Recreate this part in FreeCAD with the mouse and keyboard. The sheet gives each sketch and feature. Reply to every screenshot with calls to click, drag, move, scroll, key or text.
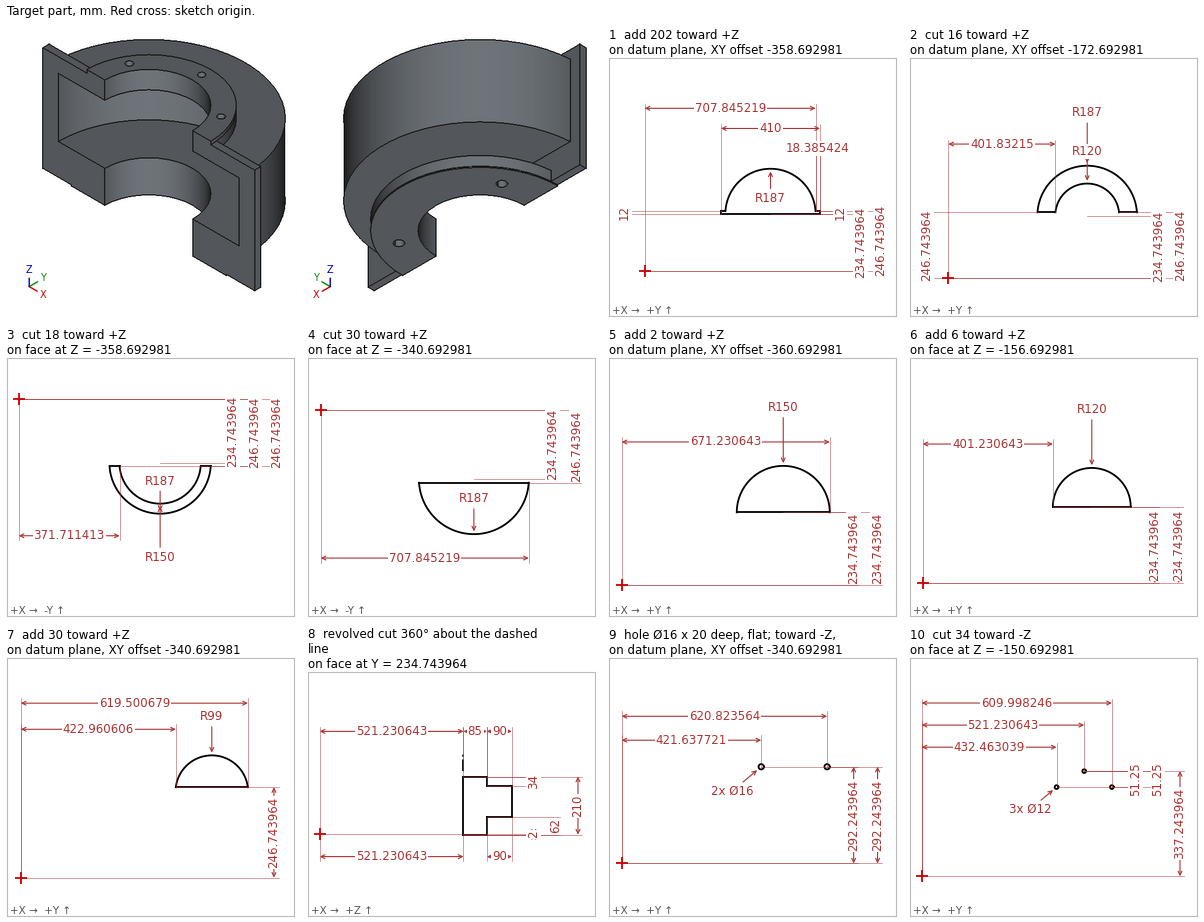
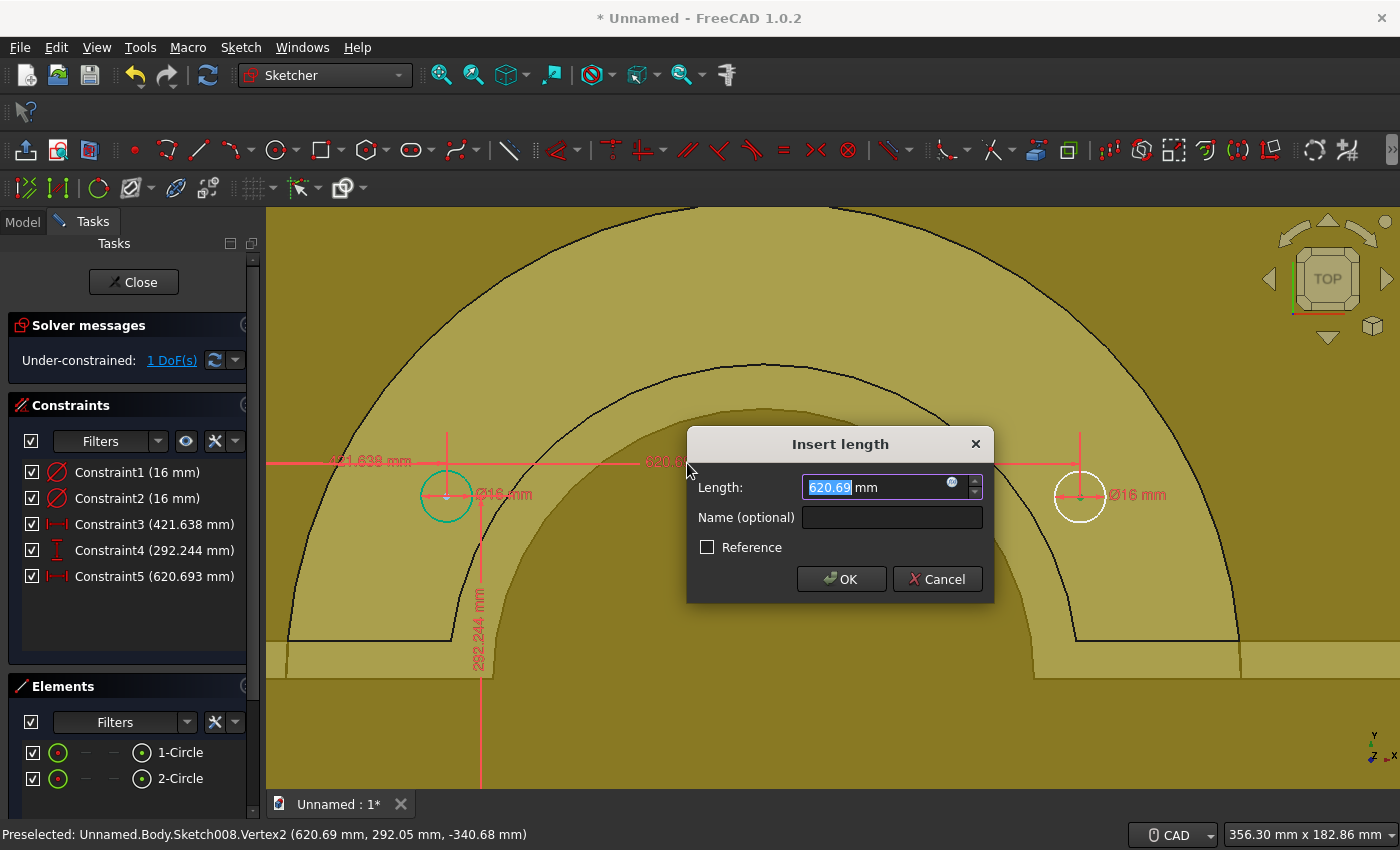
text(620.823564)
key(Return)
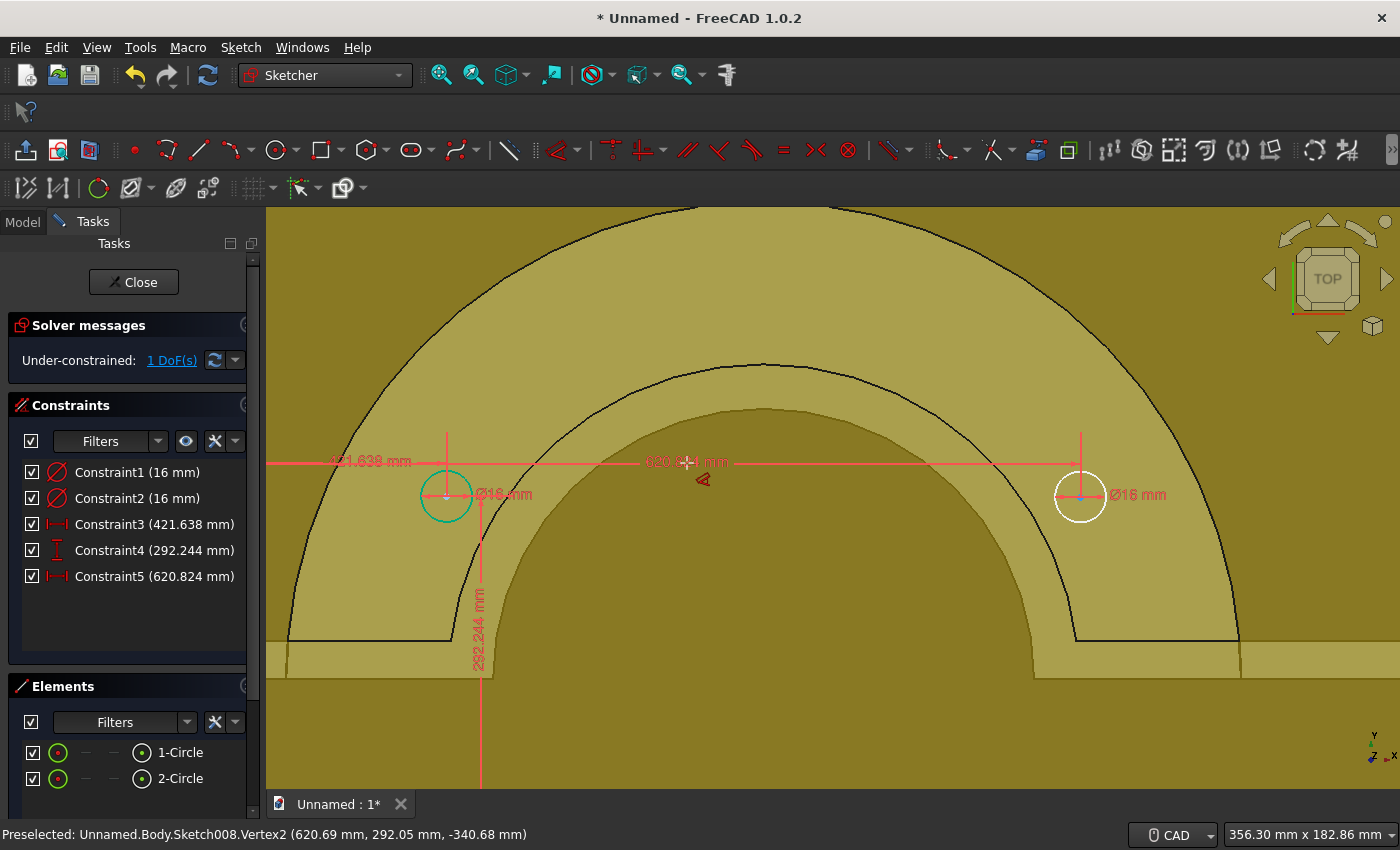
click(1081, 497)
click(1115, 629)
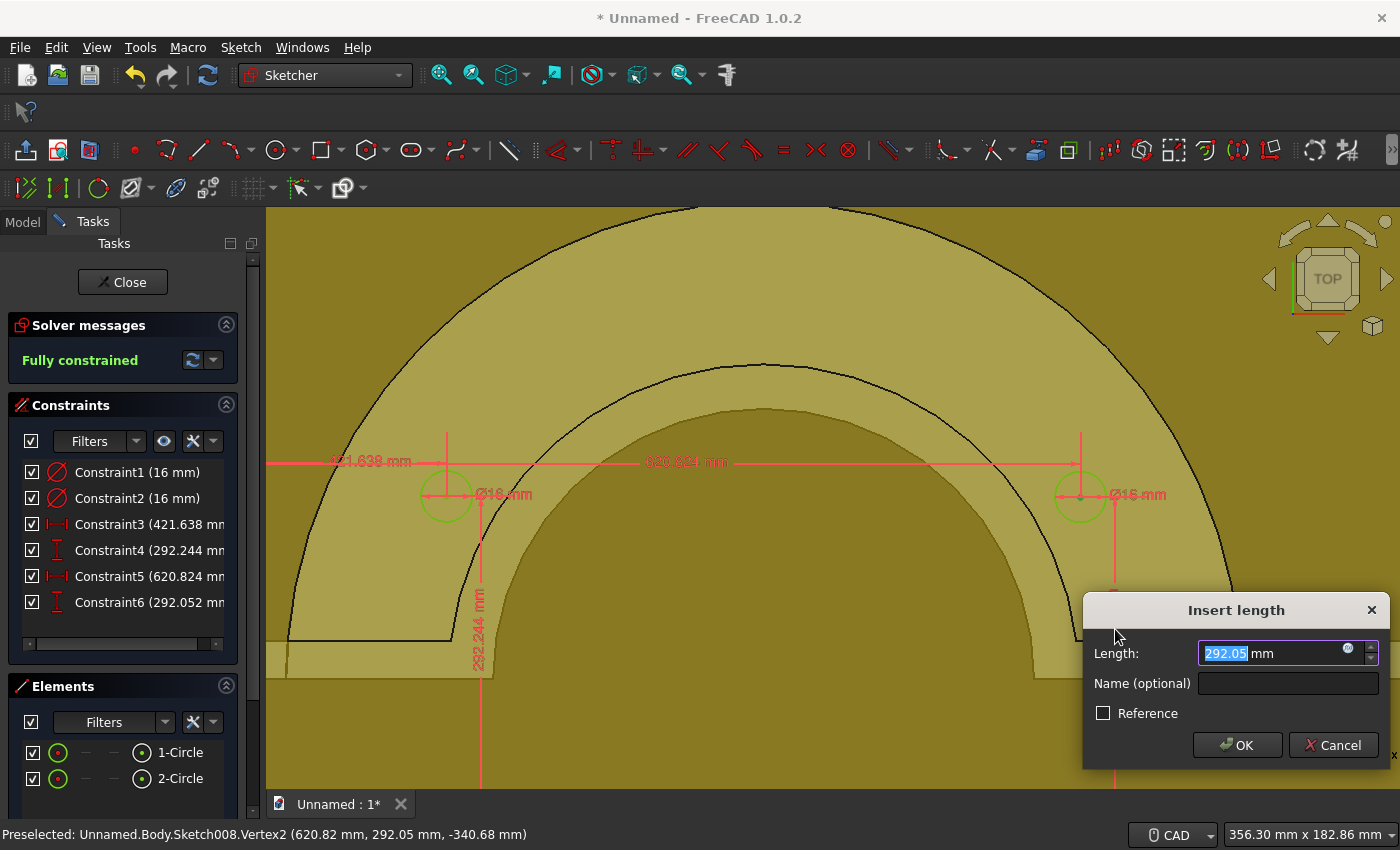
text(292.243964)
key(Return)
key(Escape)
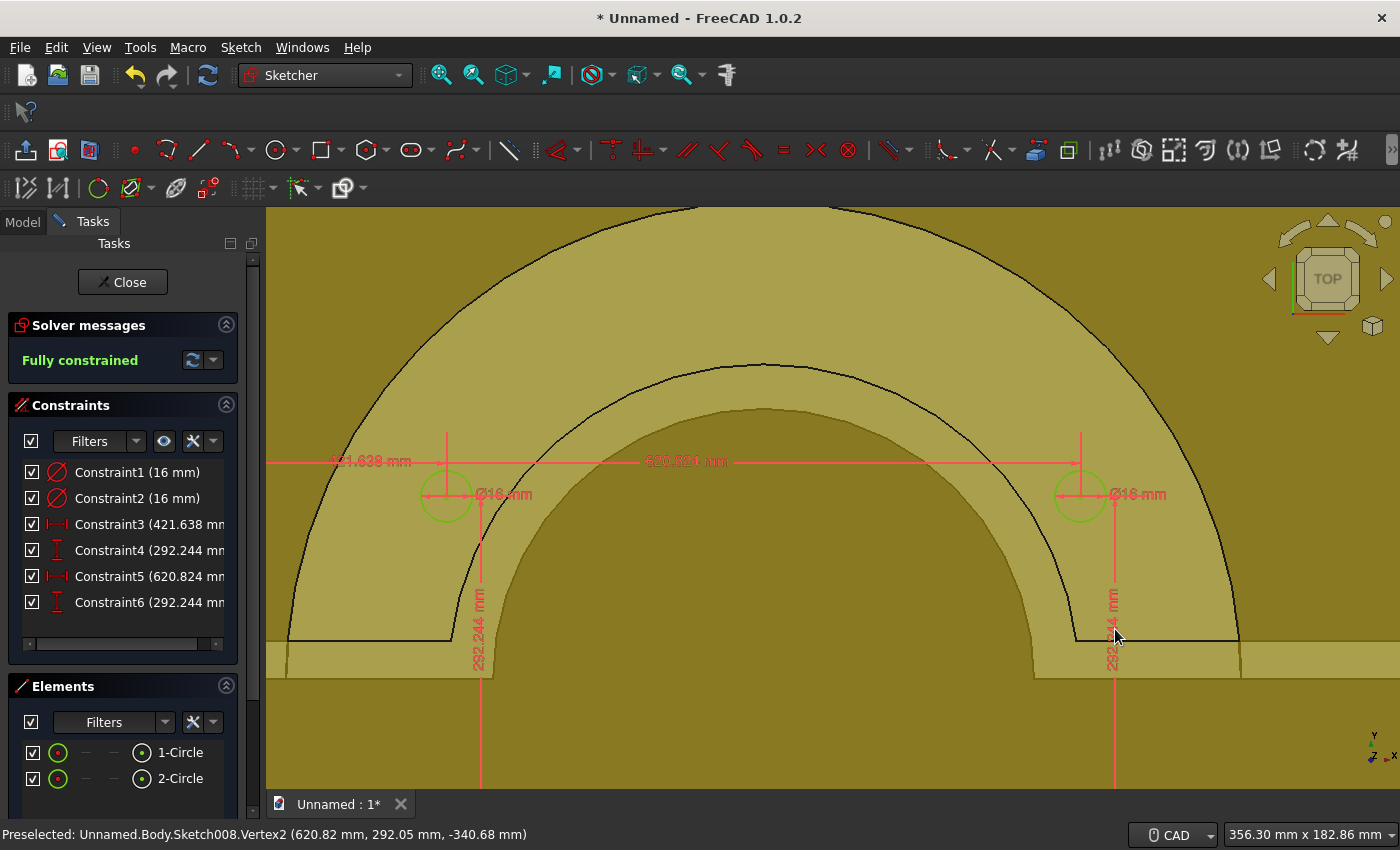
click(123, 282)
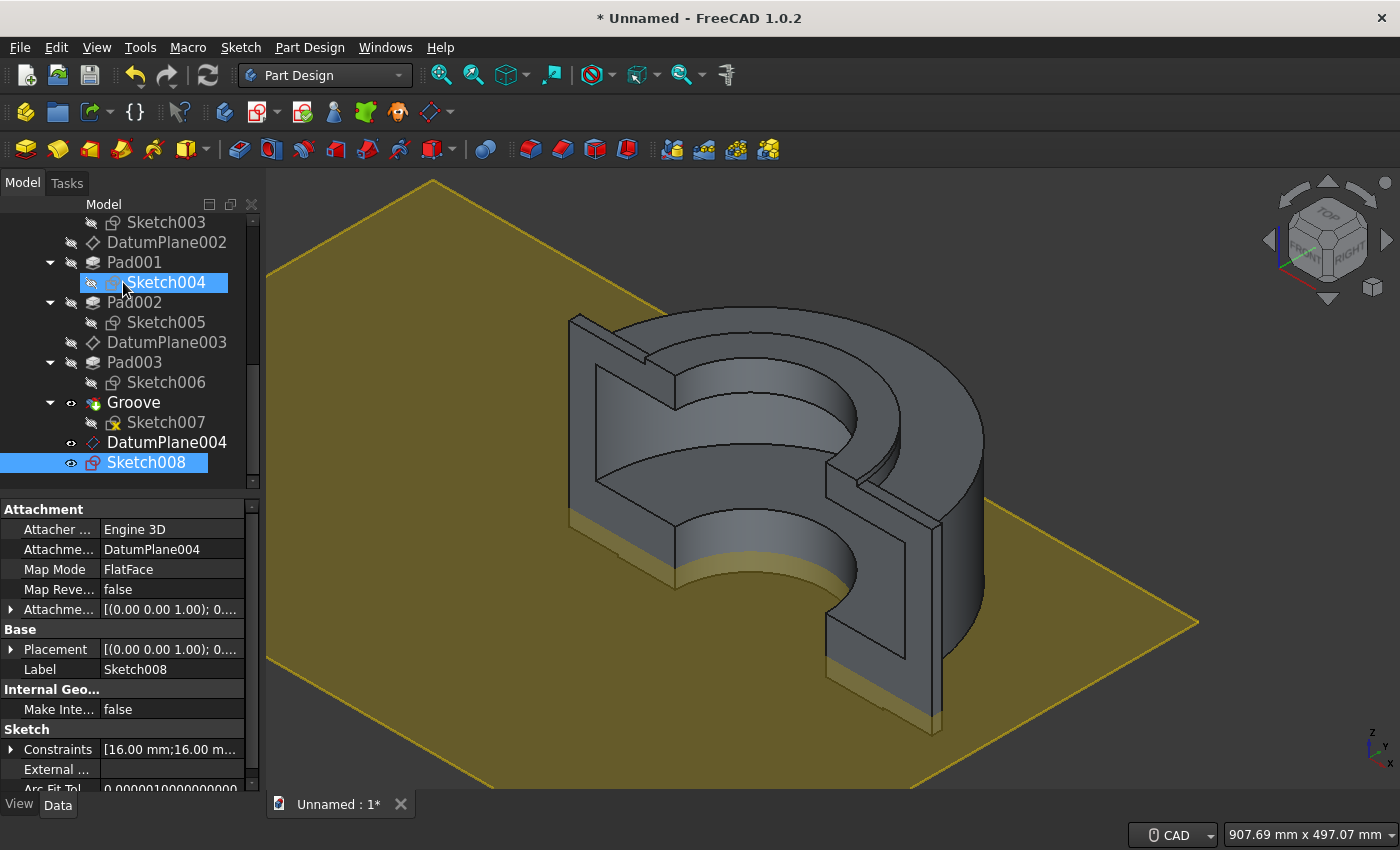
click(272, 150)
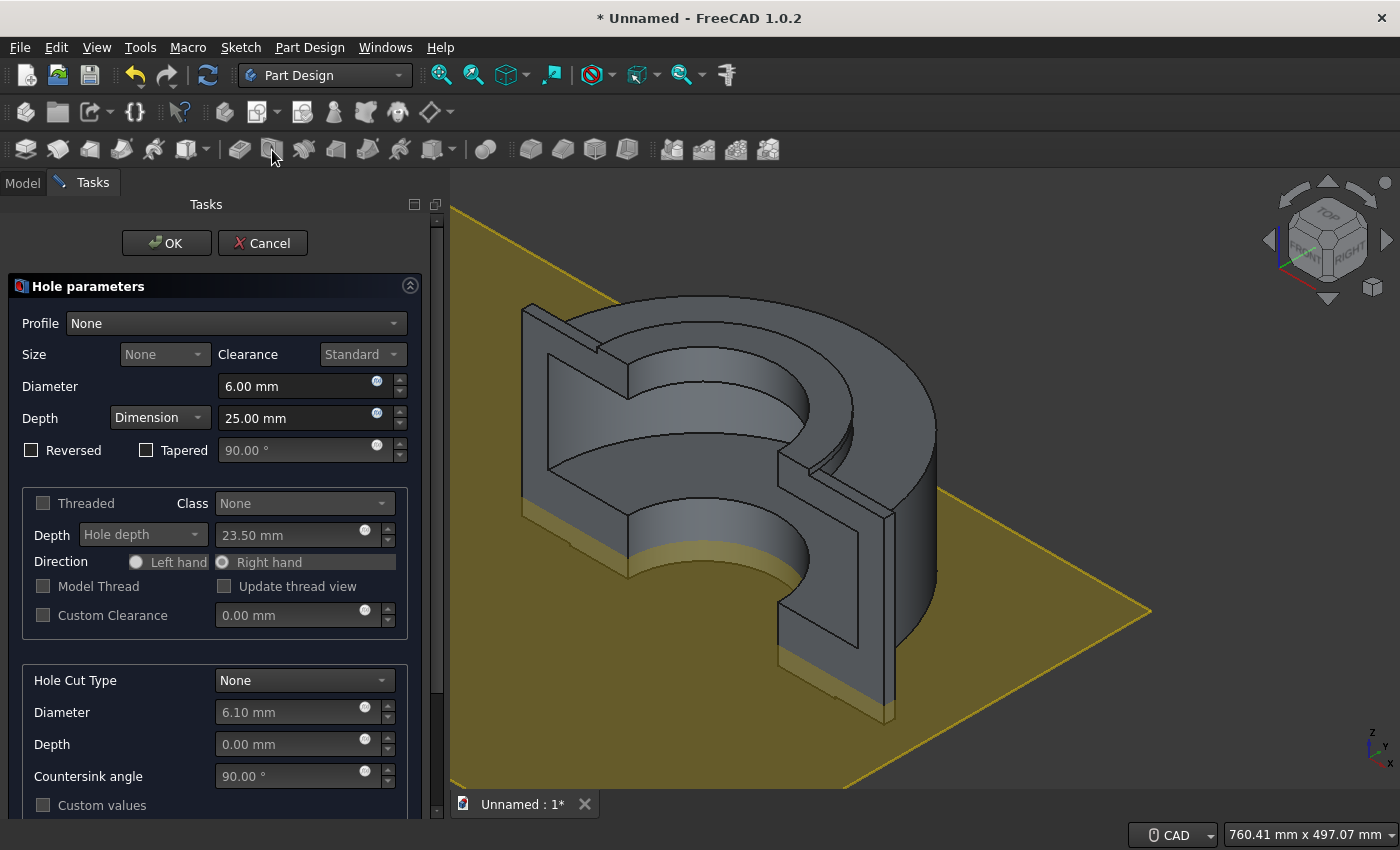
triple_click(305, 386)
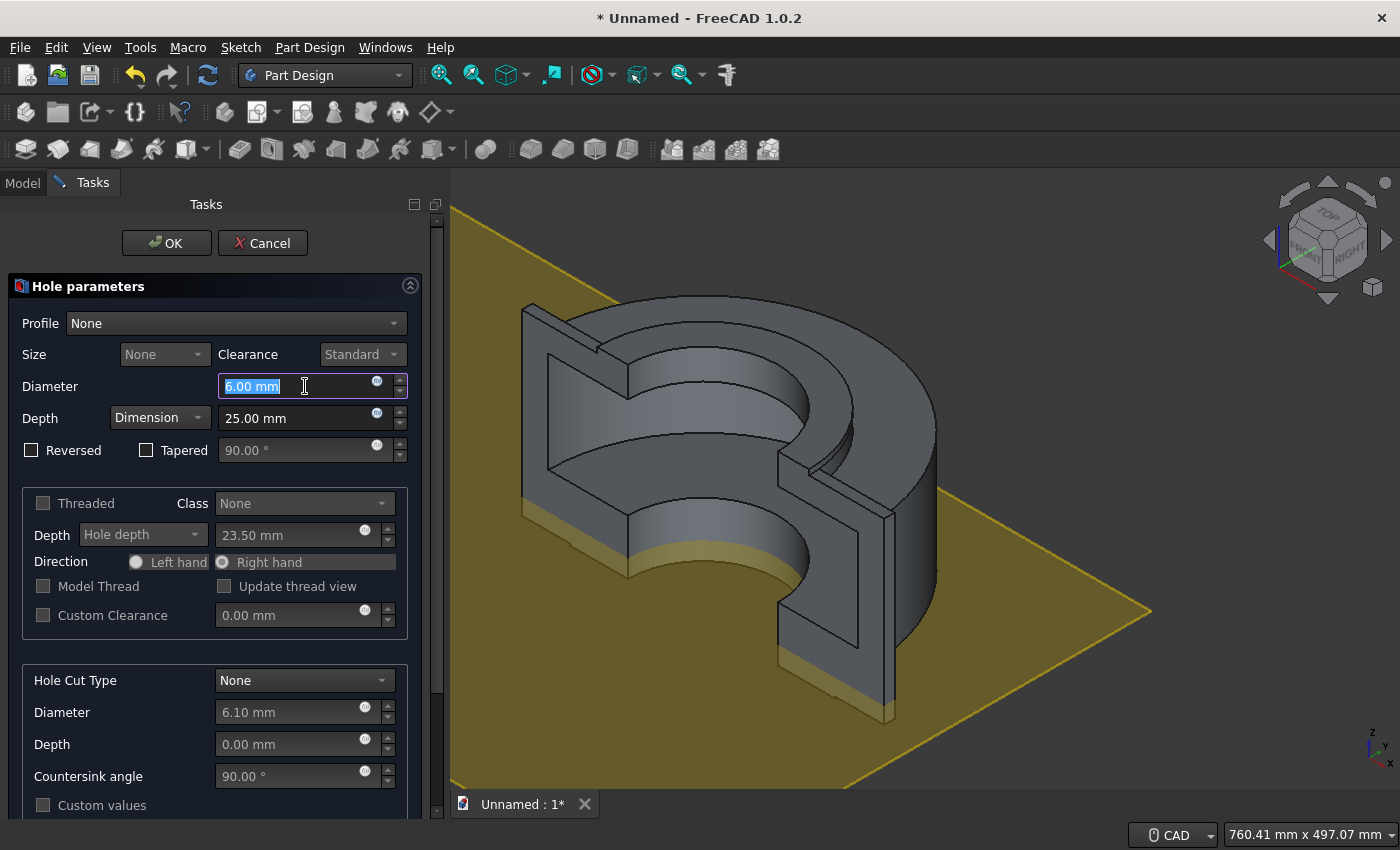
text(16)
key(Tab)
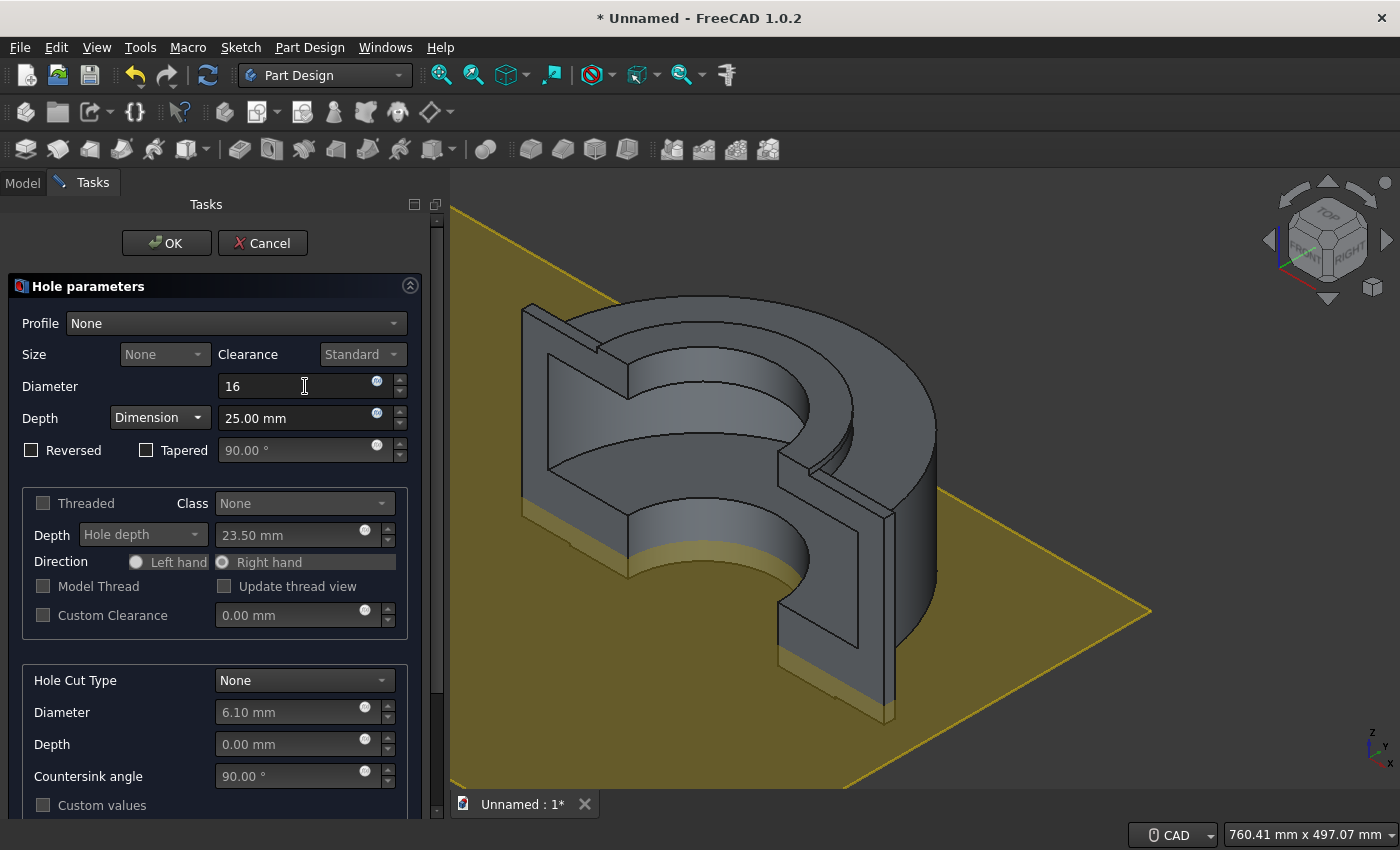
triple_click(305, 418)